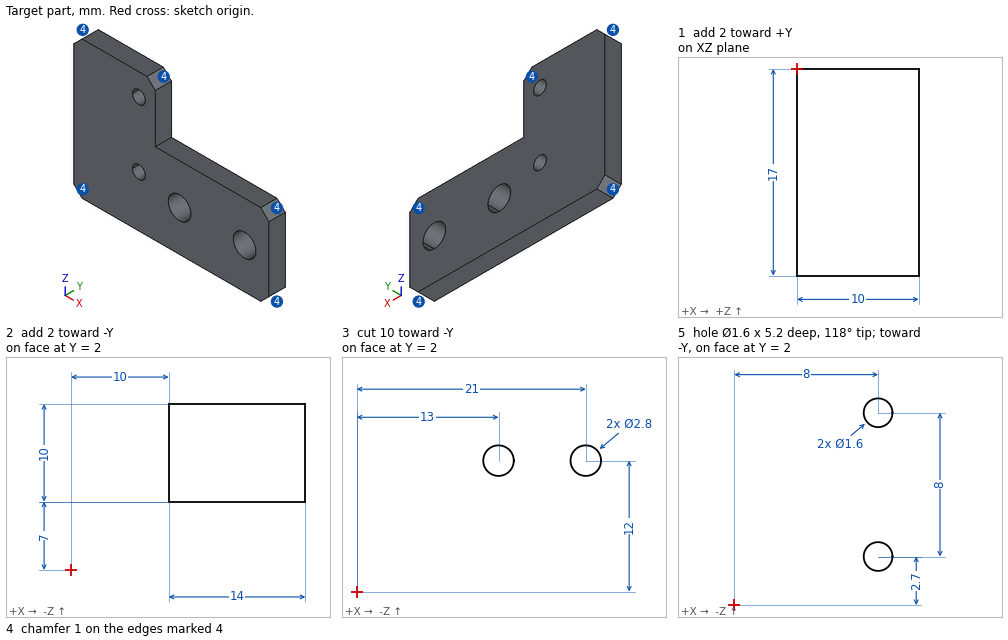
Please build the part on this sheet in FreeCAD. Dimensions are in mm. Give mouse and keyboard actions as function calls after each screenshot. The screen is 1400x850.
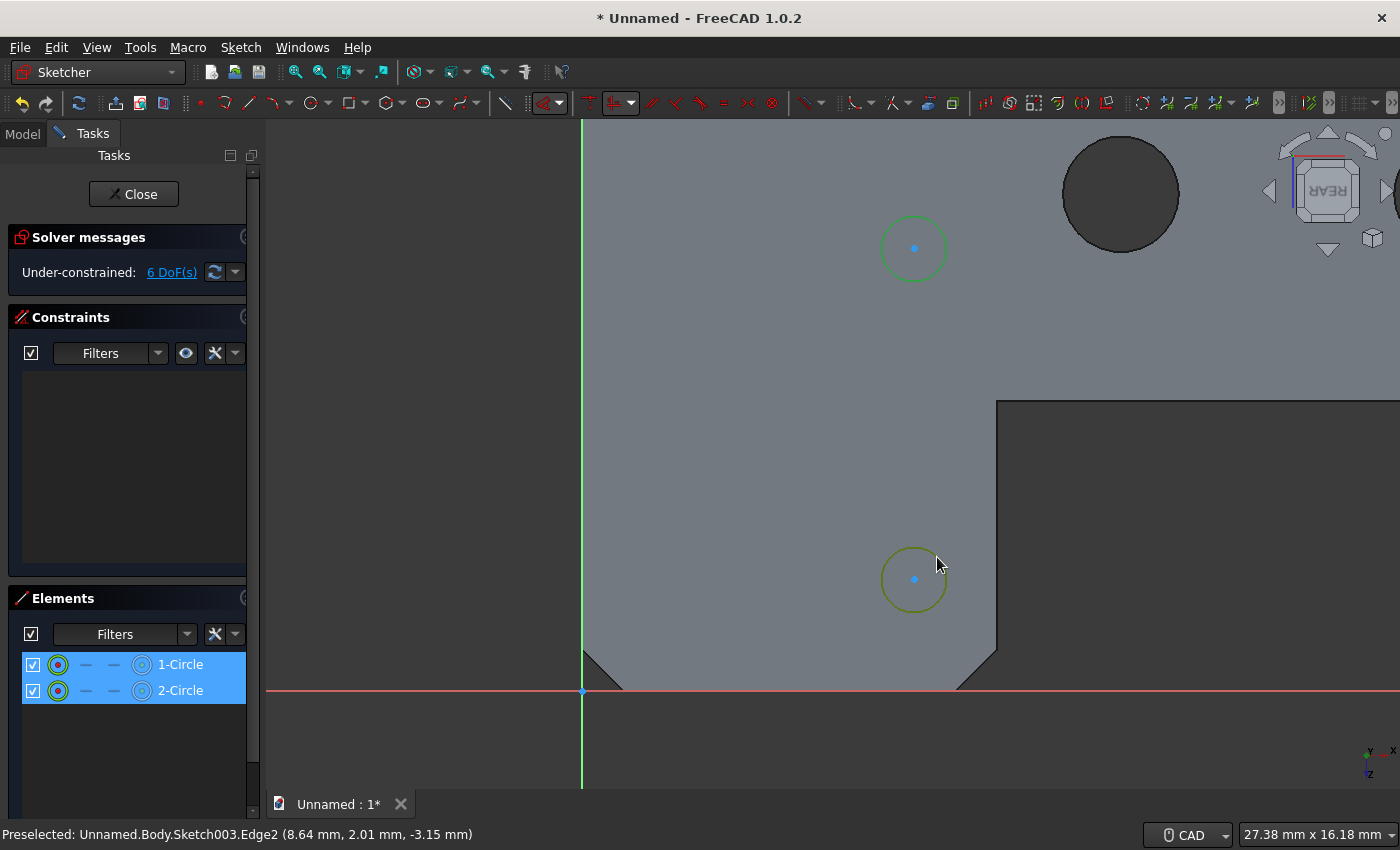
click(724, 104)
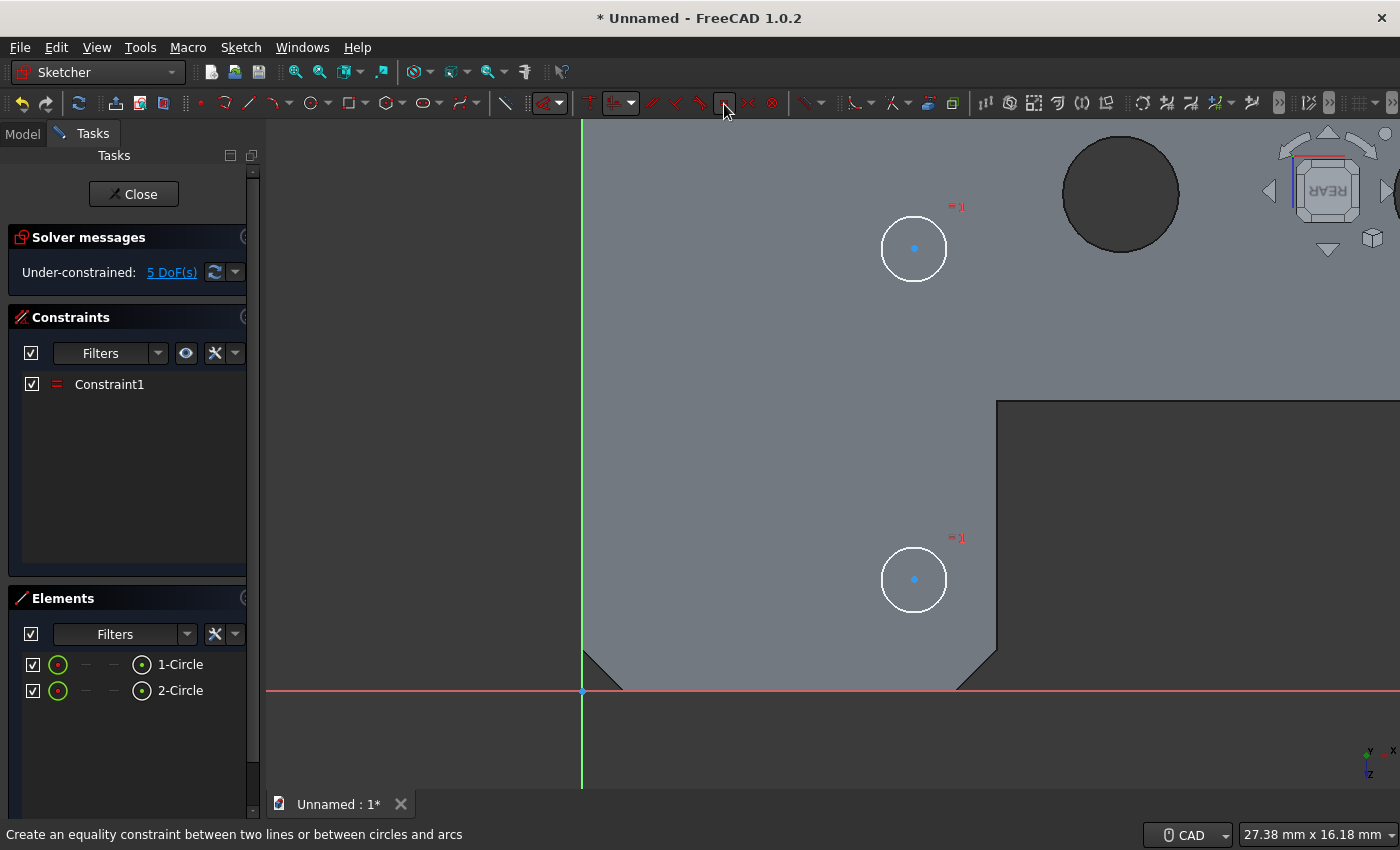
click(914, 249)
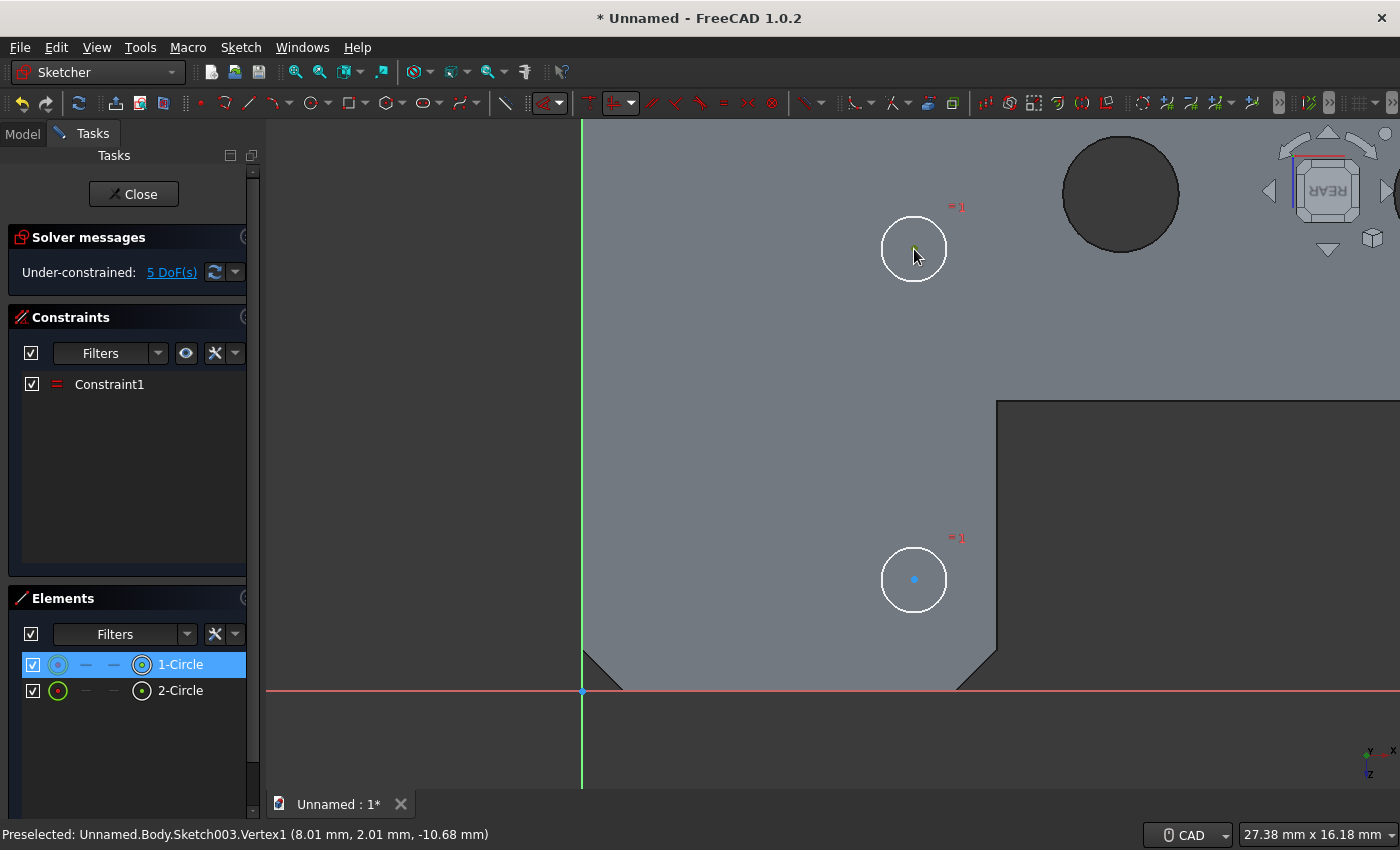
click(914, 580)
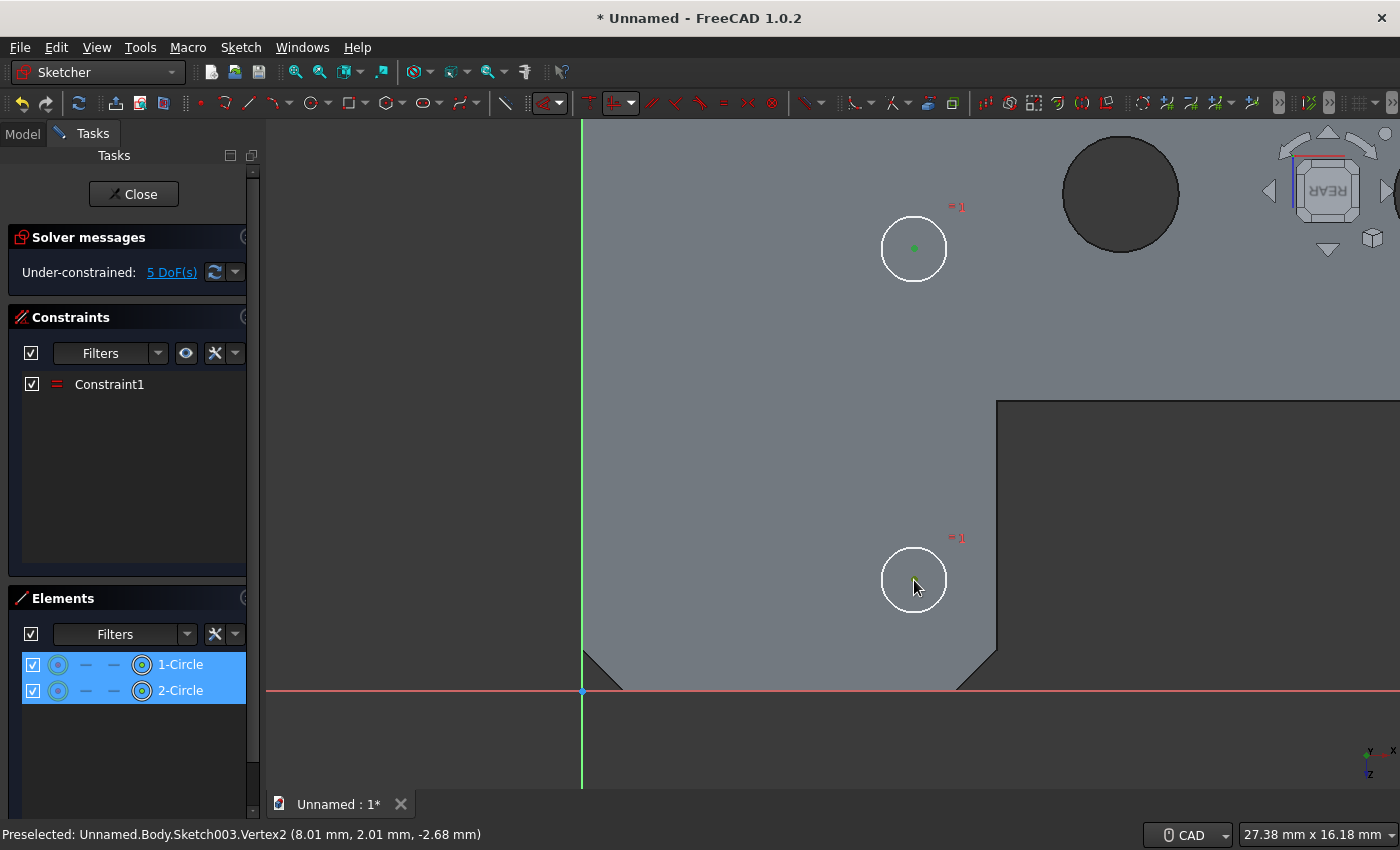
key(v)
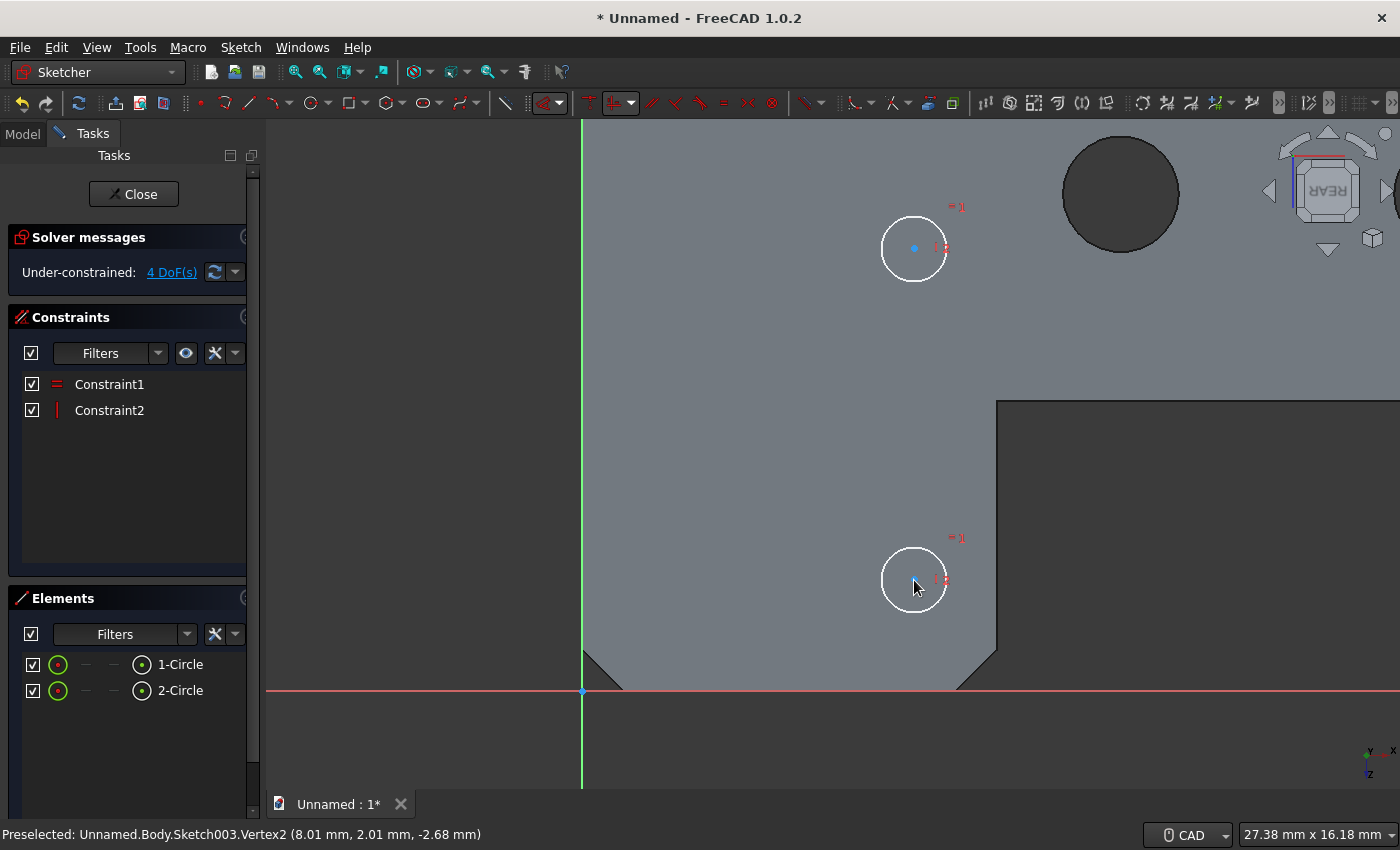
click(937, 226)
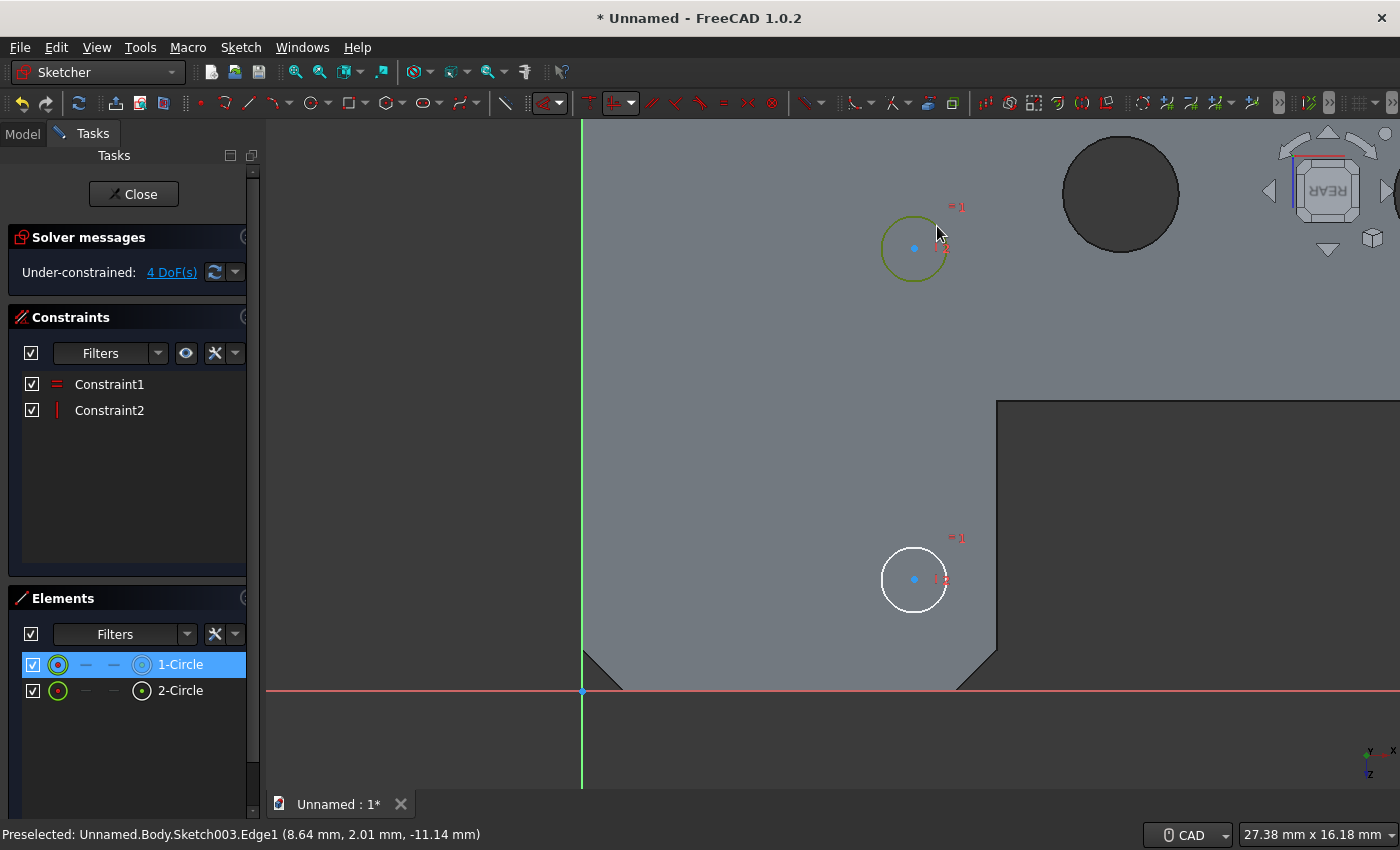
click(562, 104)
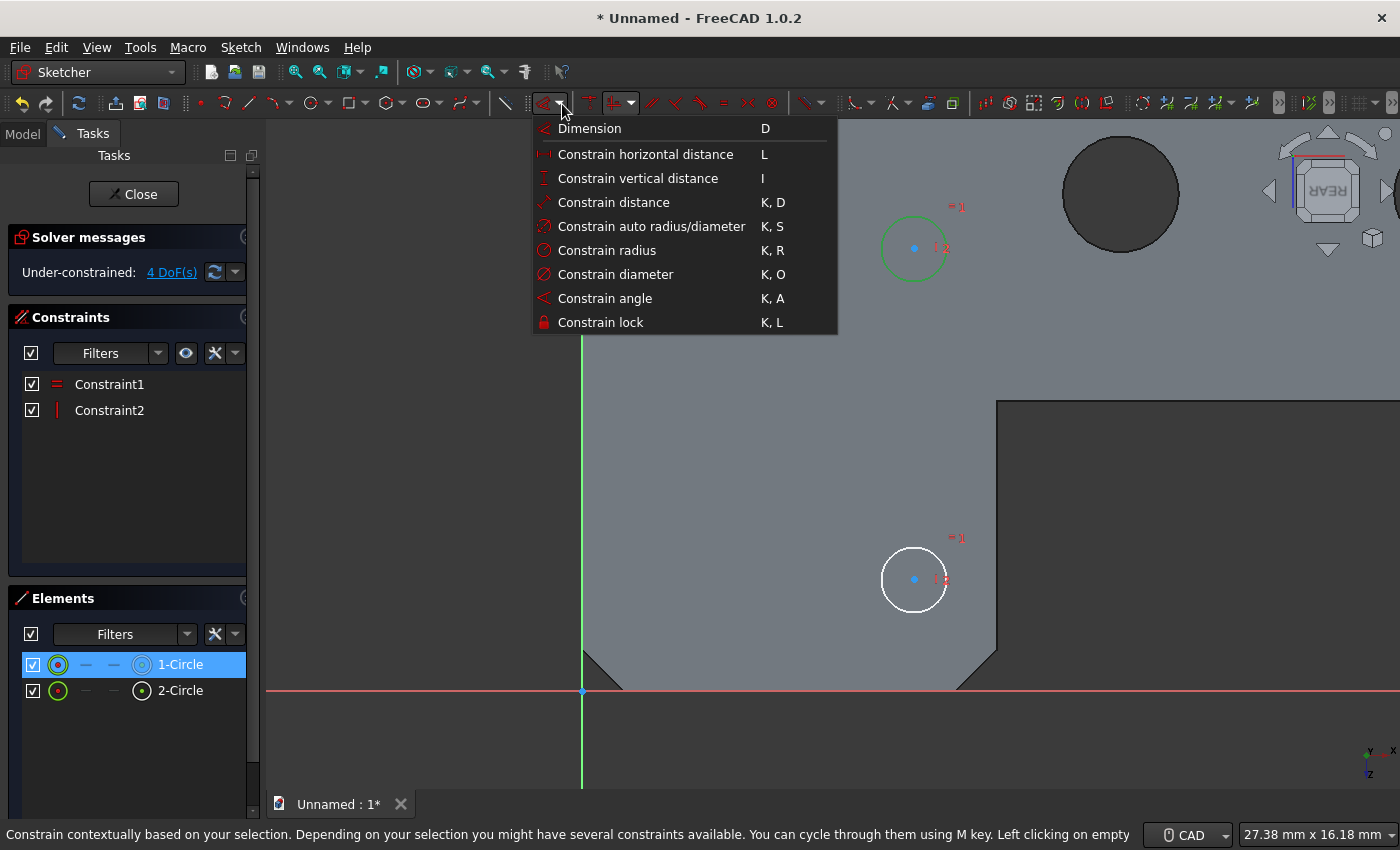
click(685, 274)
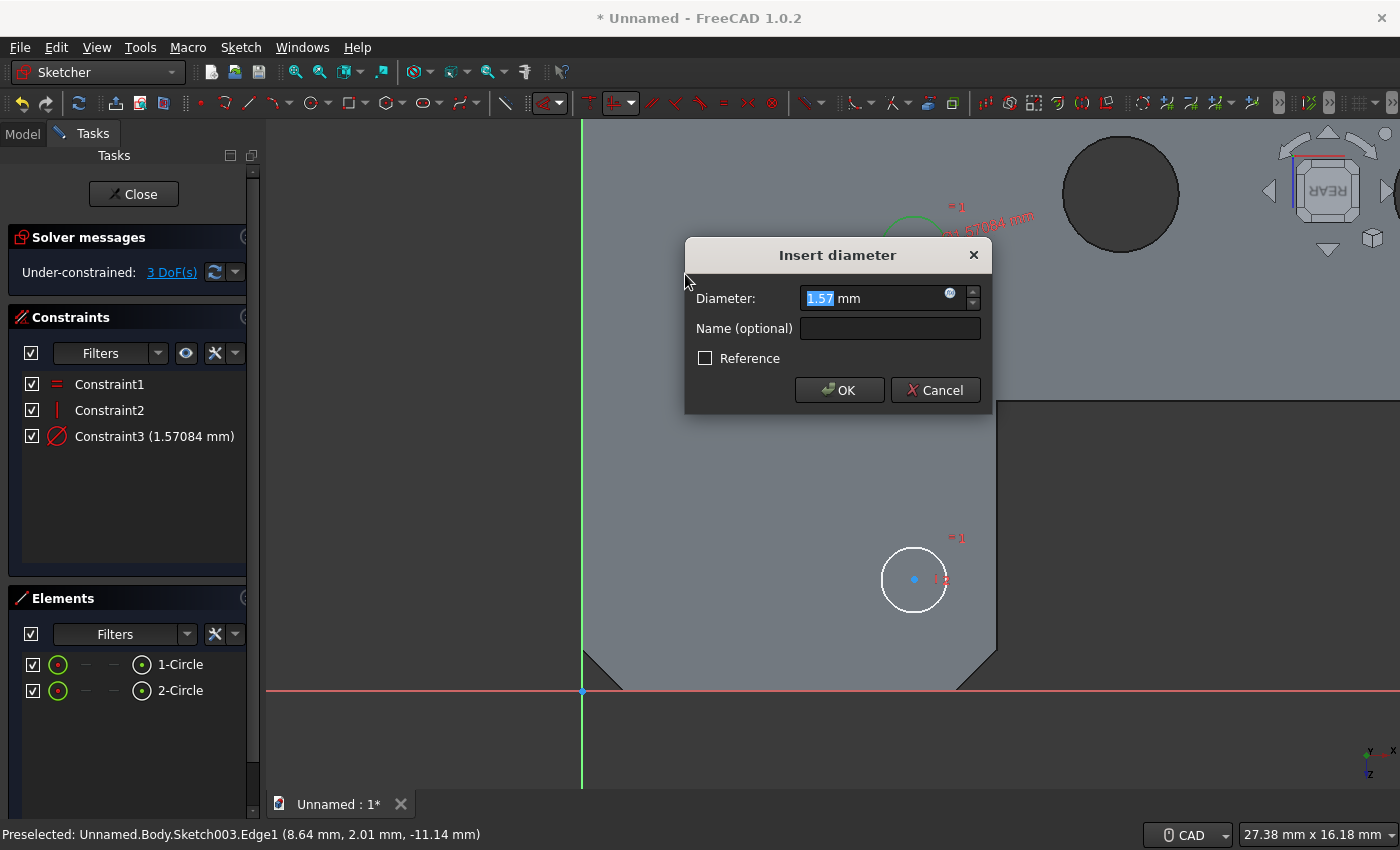
text(1.6)
key(Return)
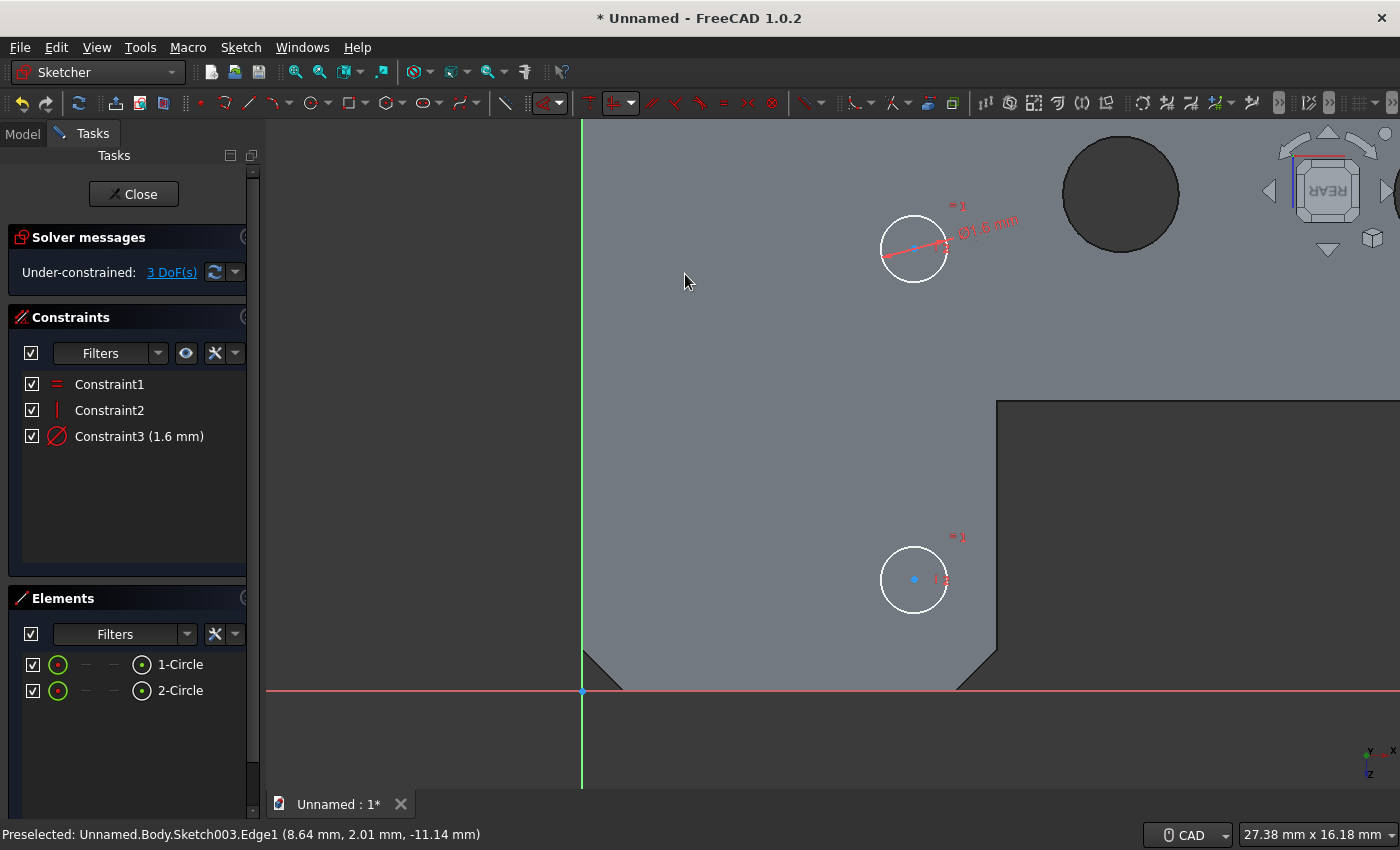
click(914, 249)